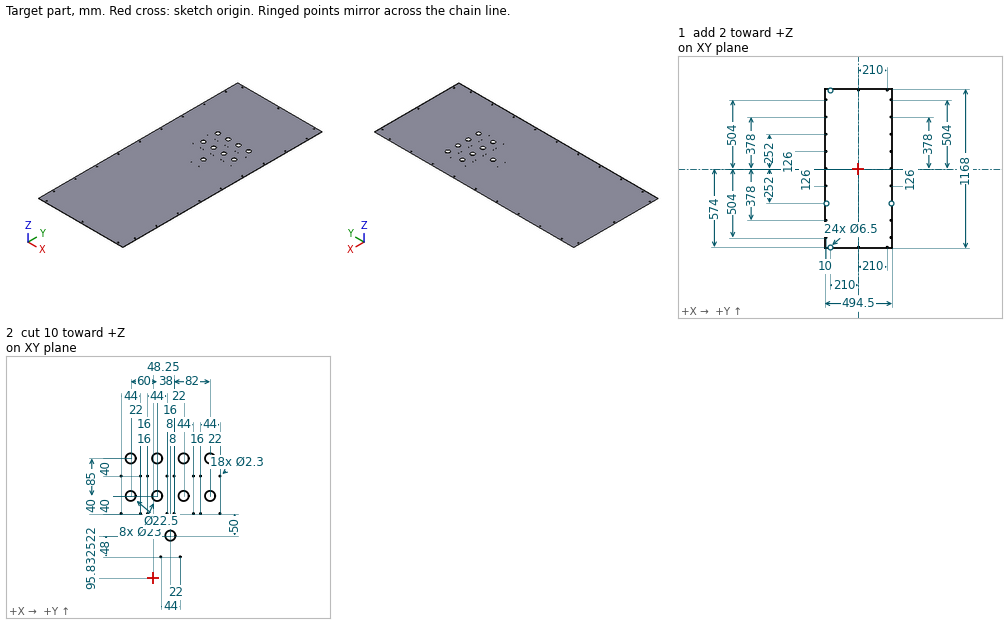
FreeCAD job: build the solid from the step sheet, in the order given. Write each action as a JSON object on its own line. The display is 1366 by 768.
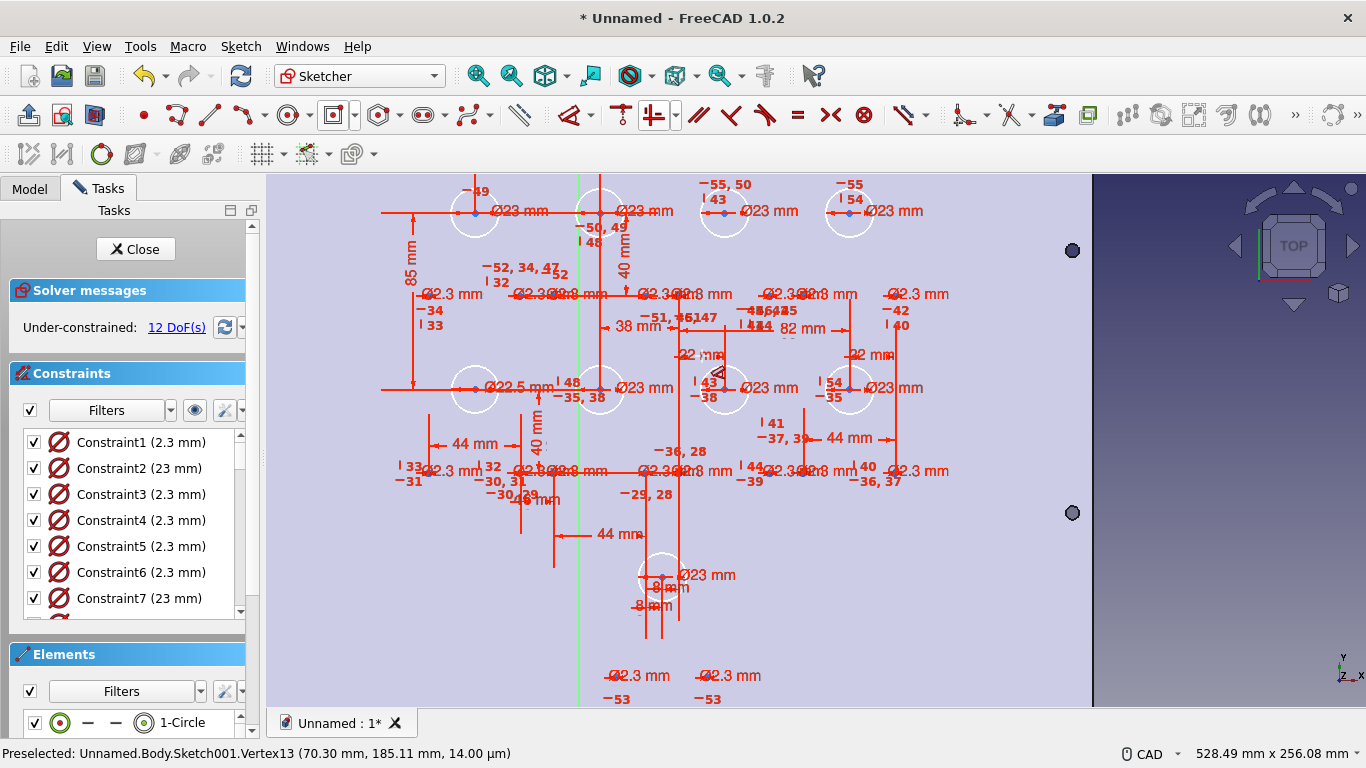
{"action": "left_click", "coordinate": [804, 473]}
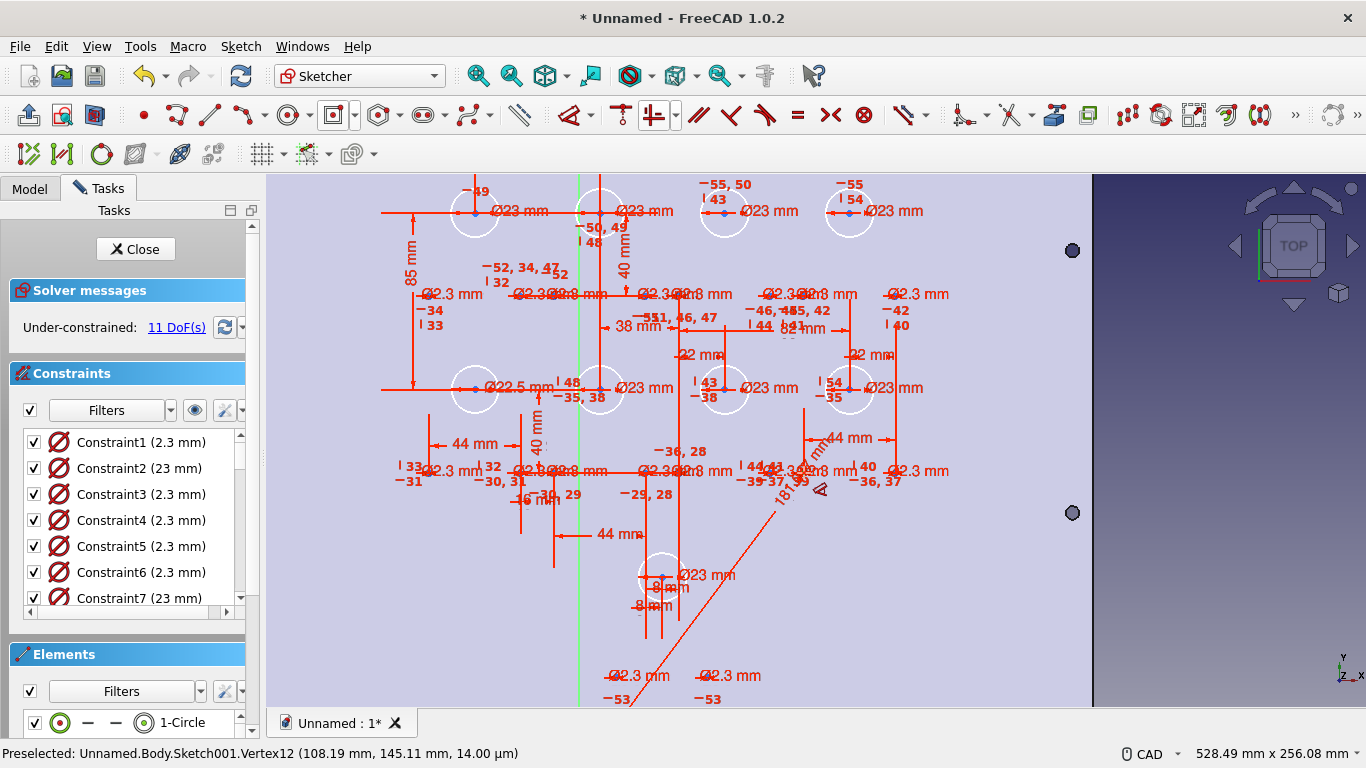
{"action": "left_click", "coordinate": [771, 473]}
{"action": "left_click", "coordinate": [780, 439]}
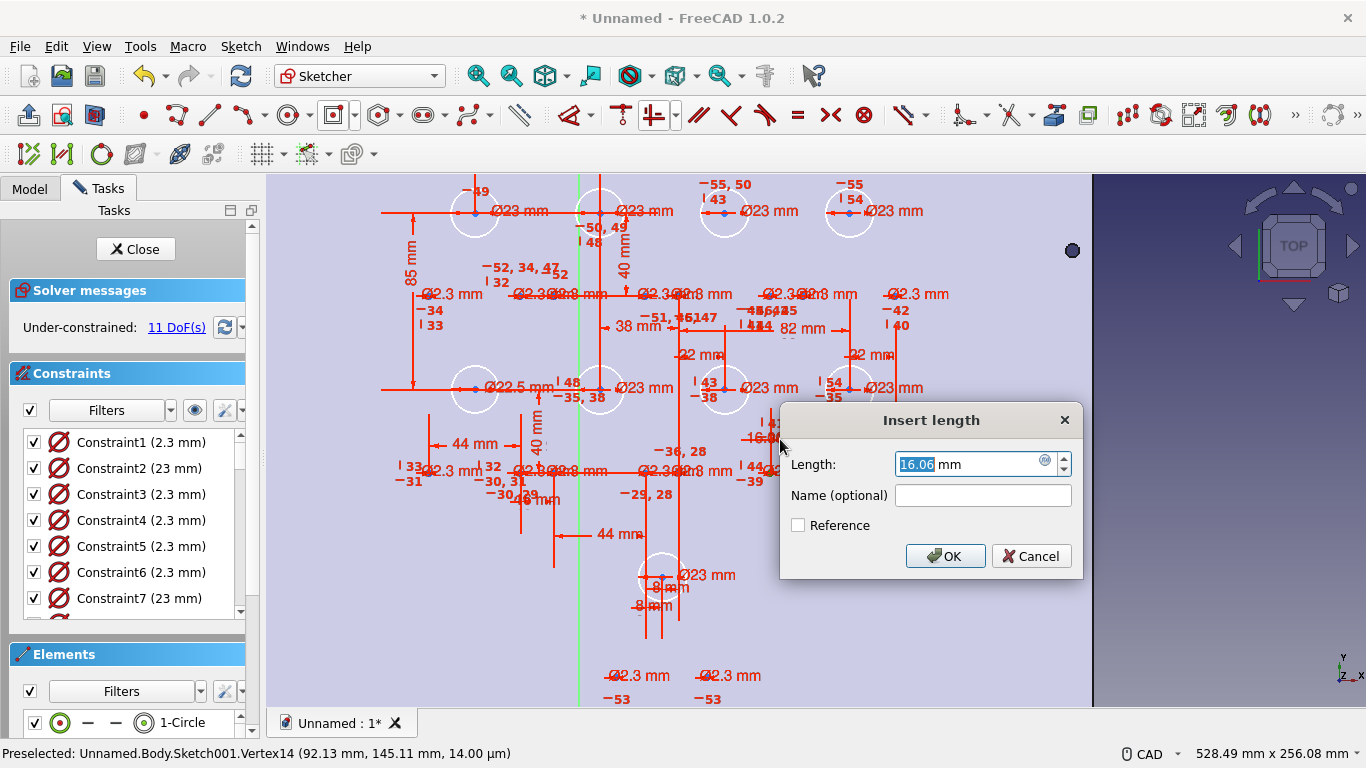
{"action": "type", "text": "16"}
{"action": "key", "text": "Return"}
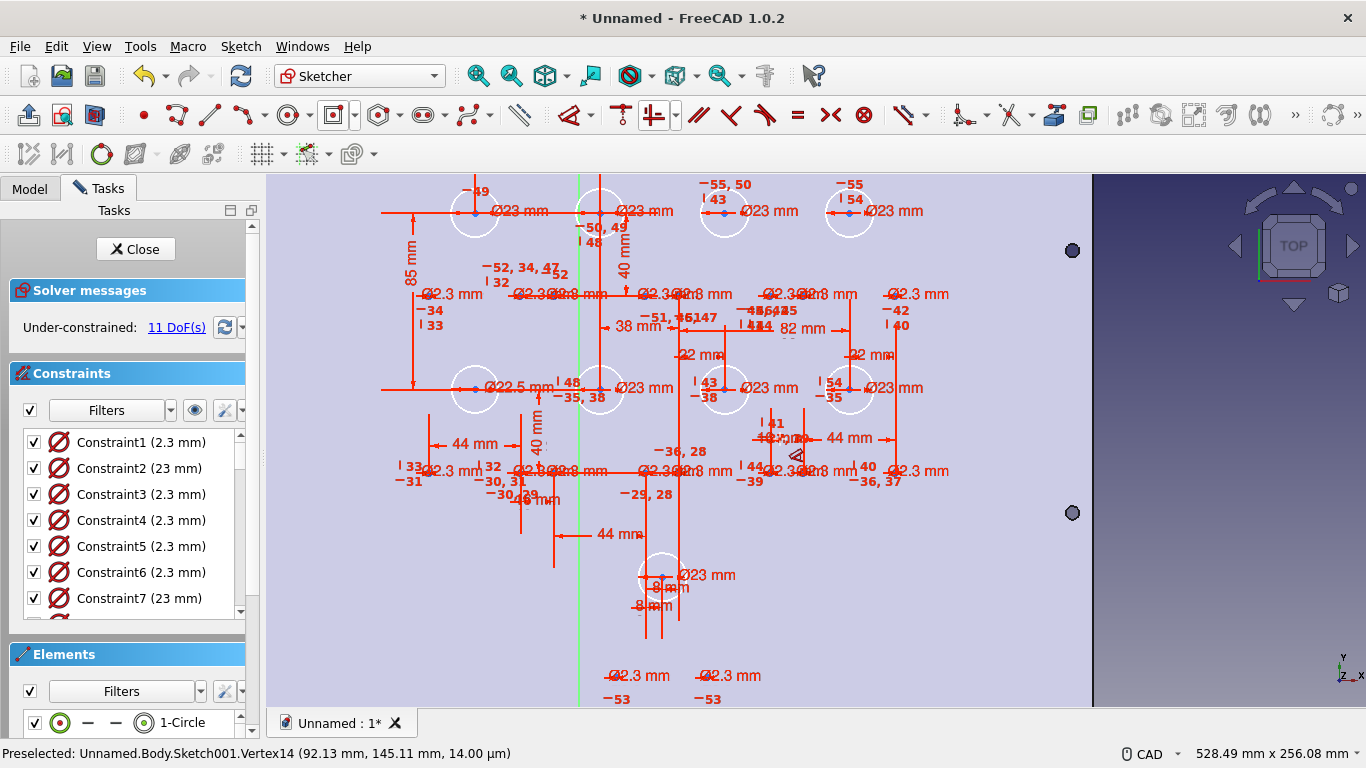
{"action": "left_click", "coordinate": [771, 296]}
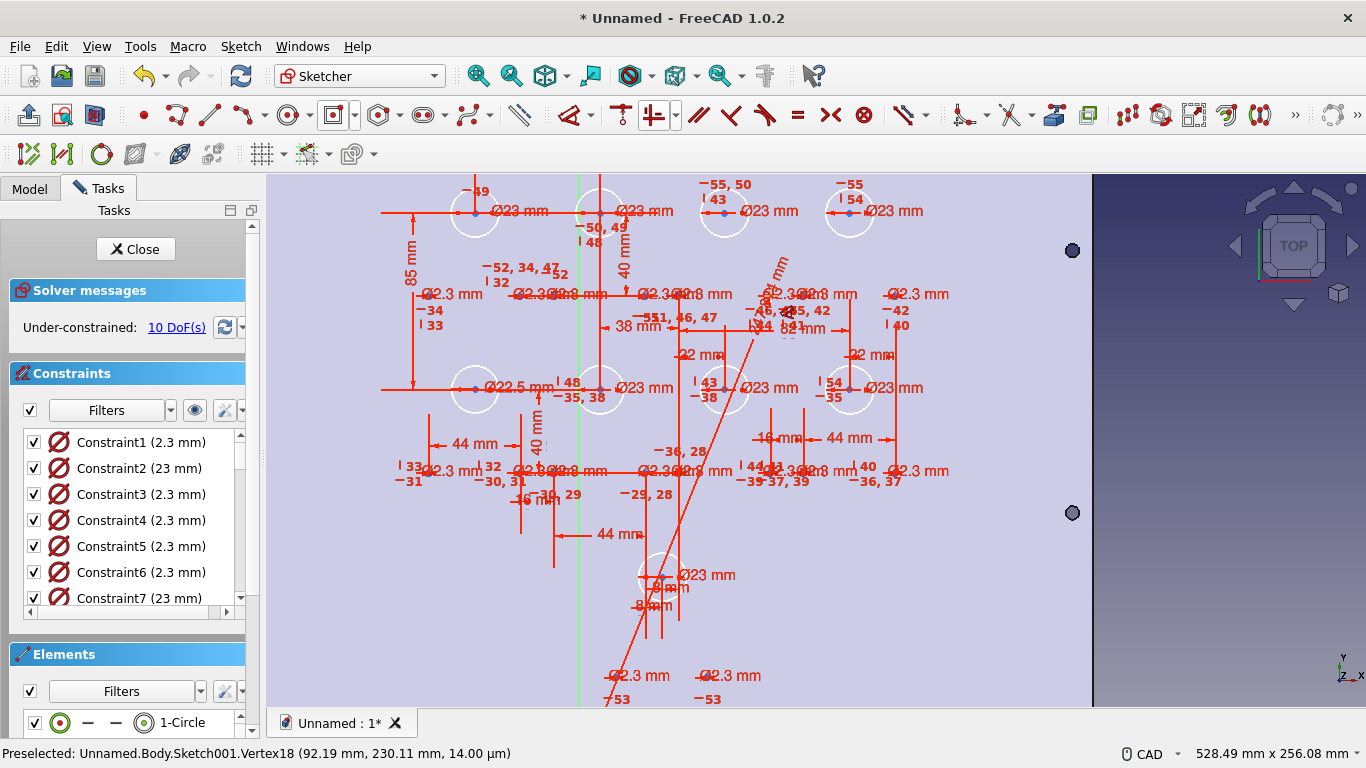
{"action": "left_click", "coordinate": [679, 296]}
{"action": "left_click", "coordinate": [725, 262]}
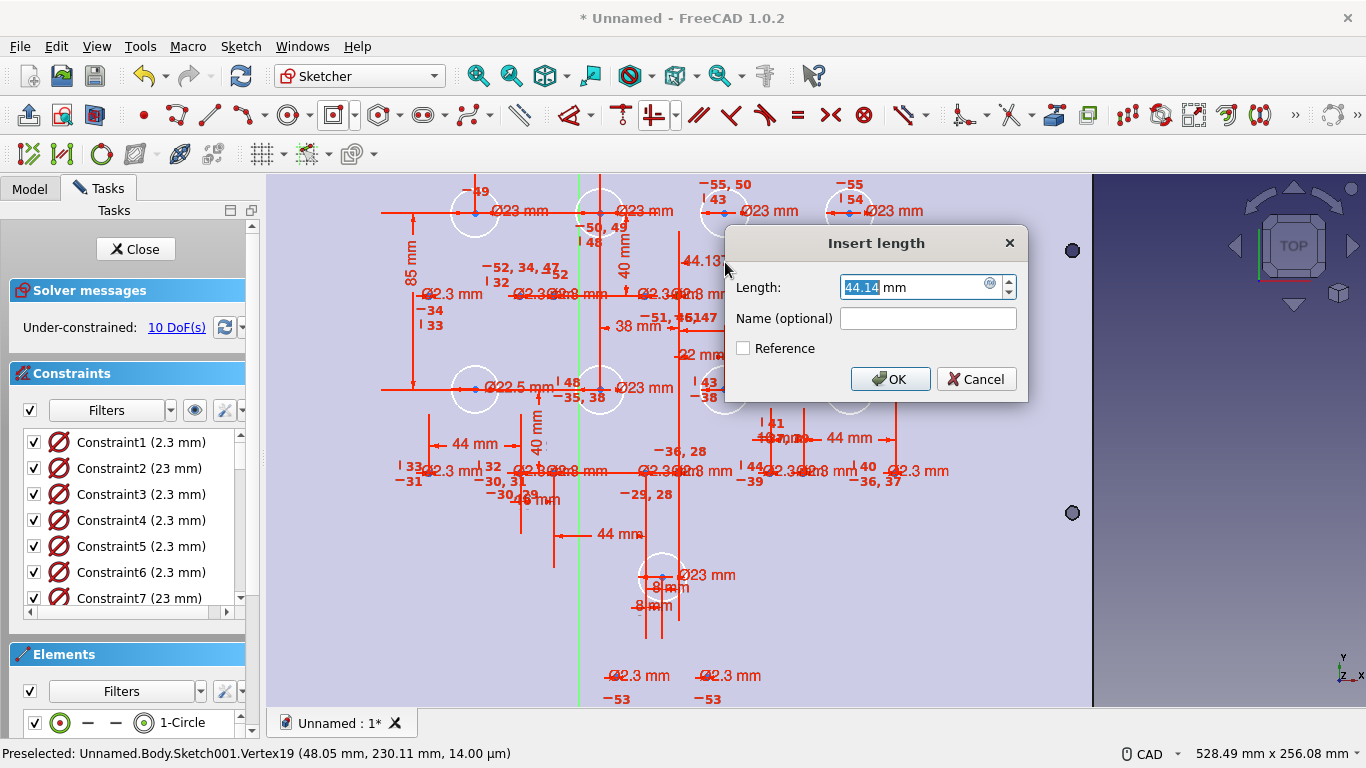
{"action": "type", "text": "44"}
{"action": "key", "text": "Return"}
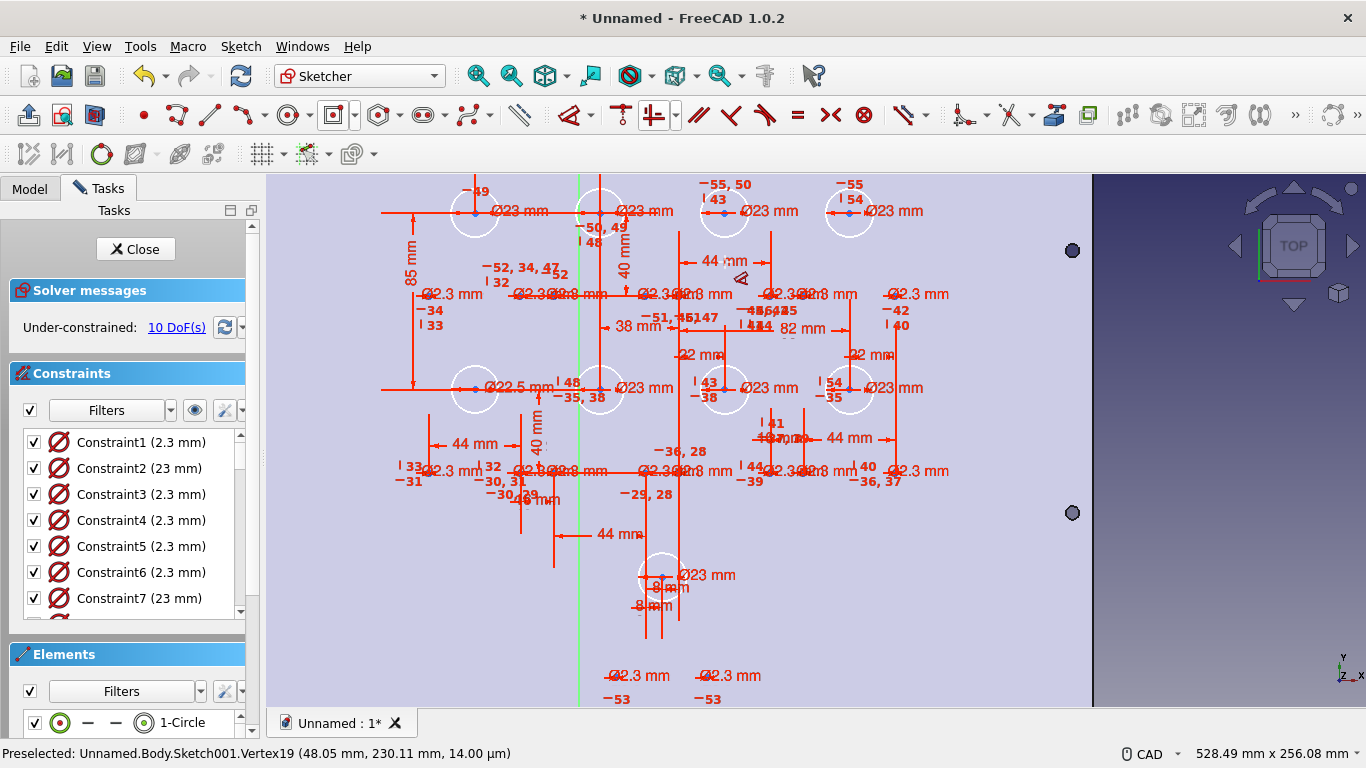
{"action": "left_click", "coordinate": [679, 296]}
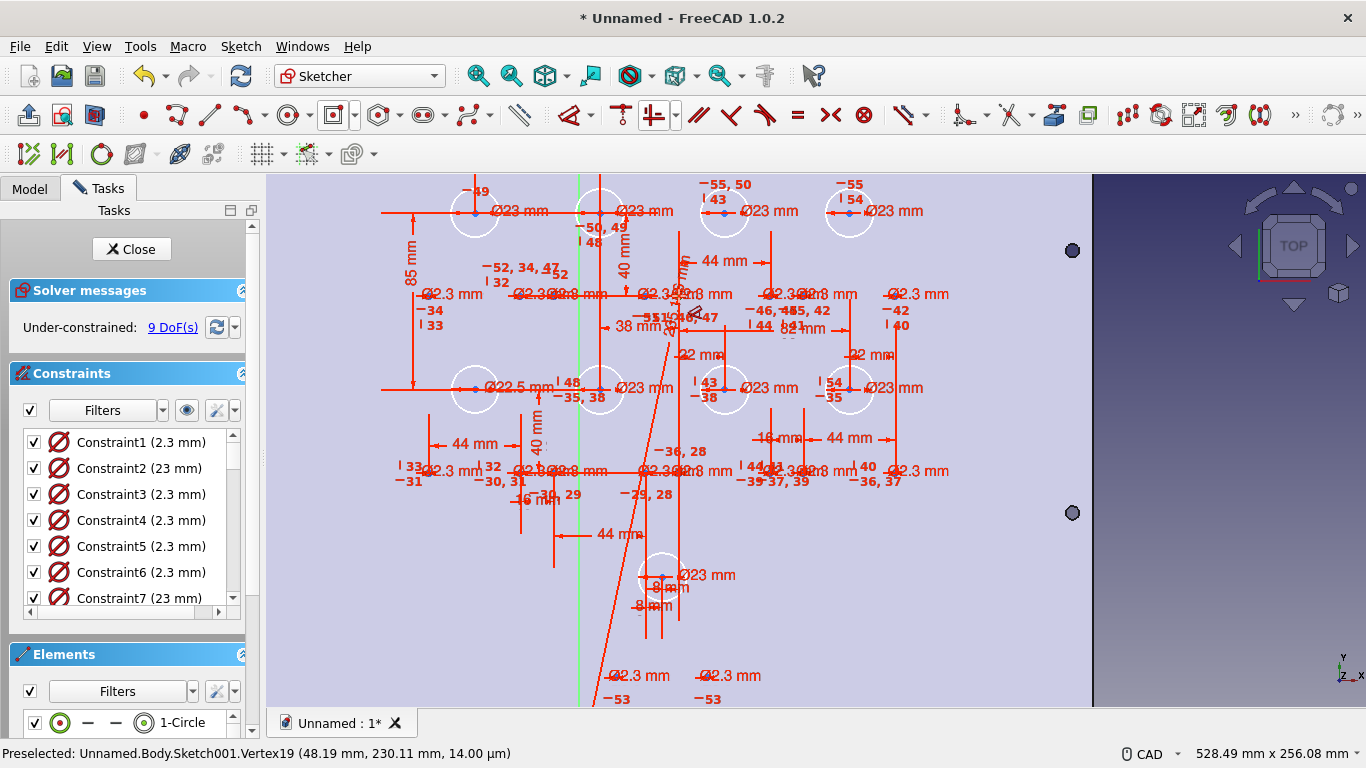
{"action": "left_click", "coordinate": [645, 296]}
{"action": "left_click", "coordinate": [662, 214]}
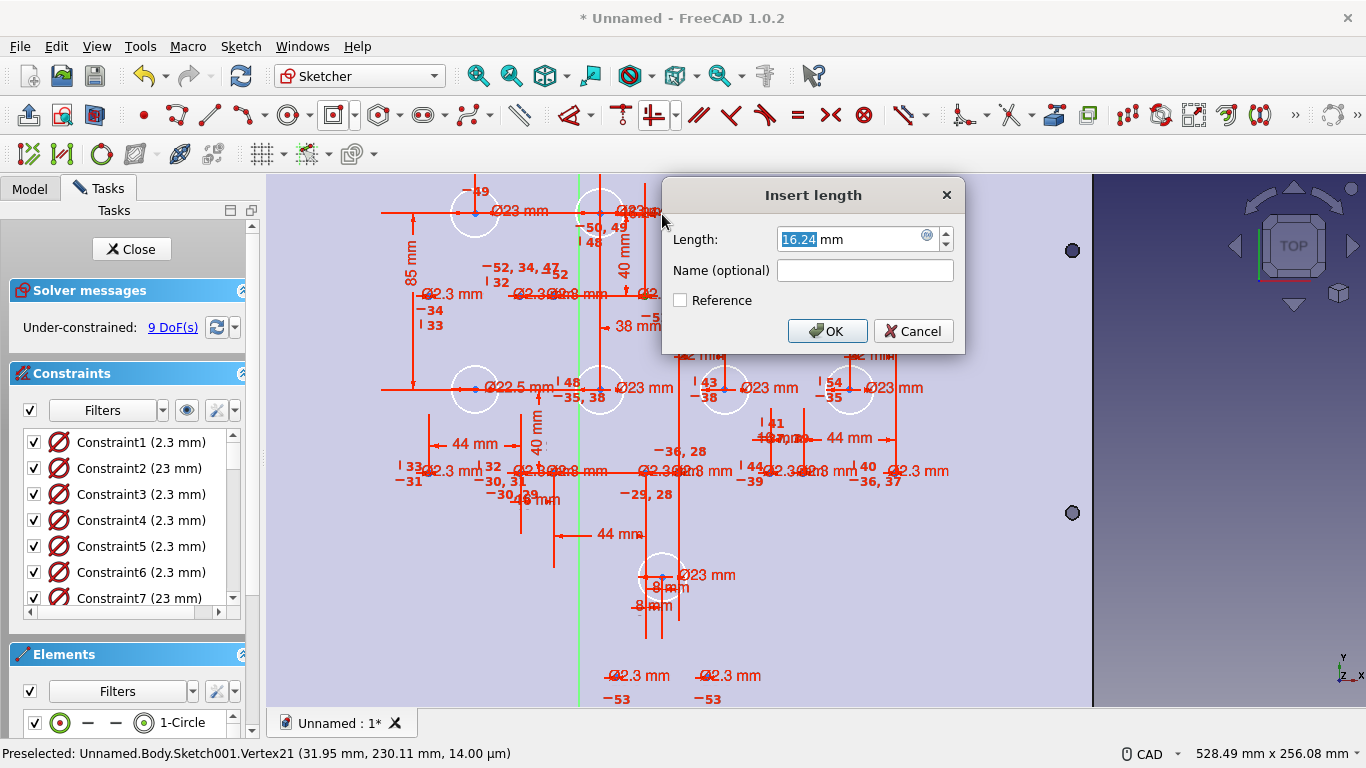
{"action": "type", "text": "16"}
{"action": "key", "text": "Return"}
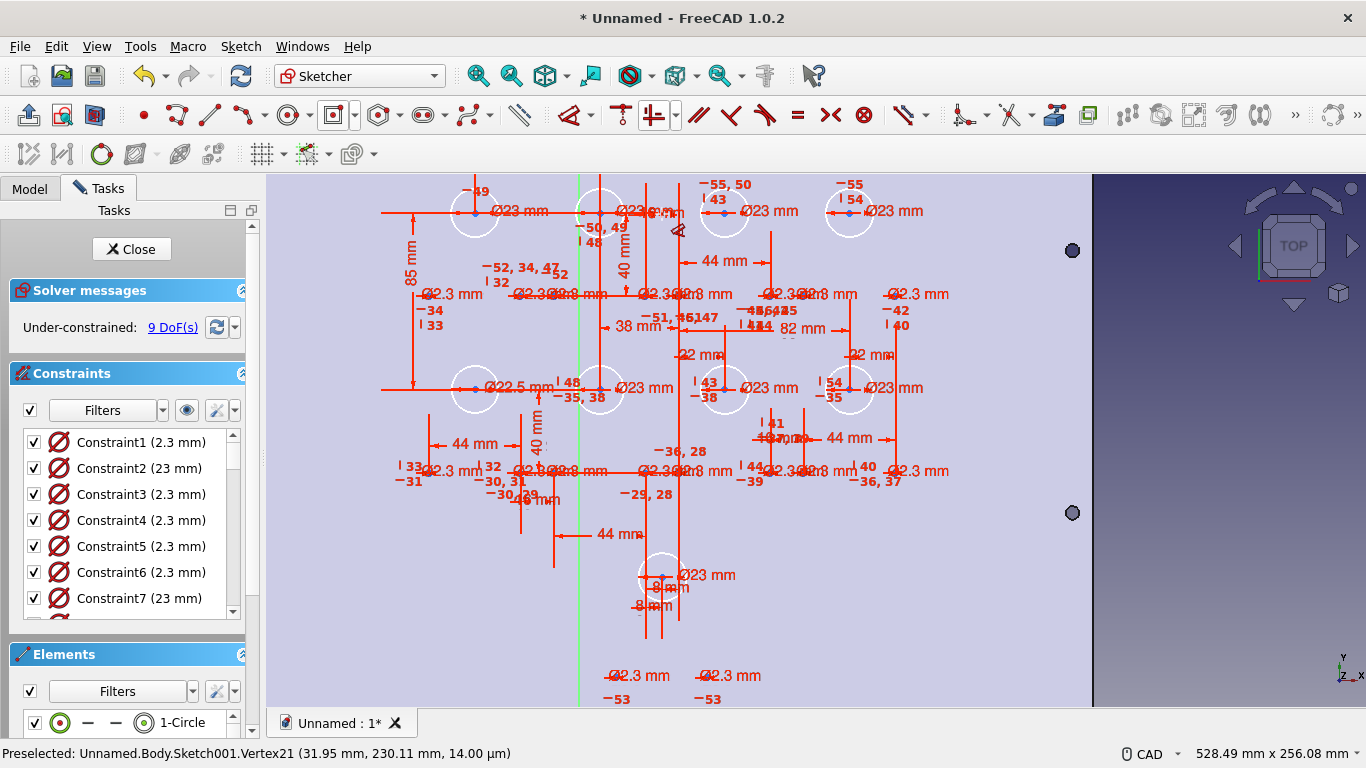
{"action": "left_click", "coordinate": [521, 296]}